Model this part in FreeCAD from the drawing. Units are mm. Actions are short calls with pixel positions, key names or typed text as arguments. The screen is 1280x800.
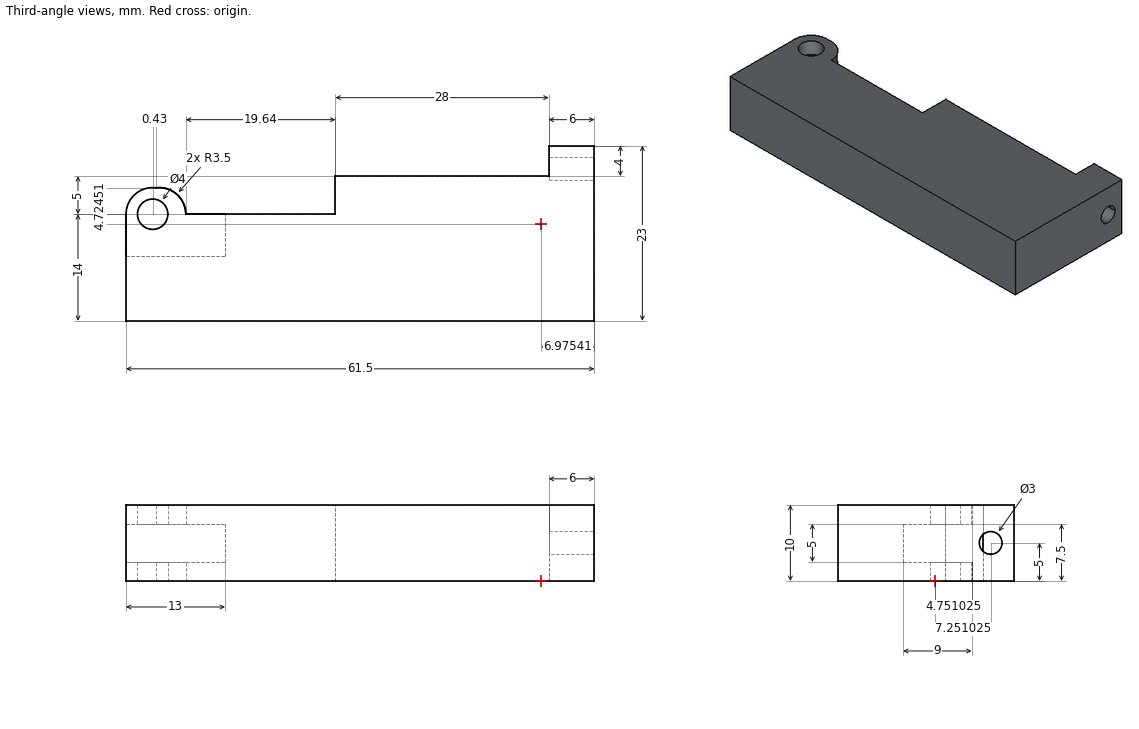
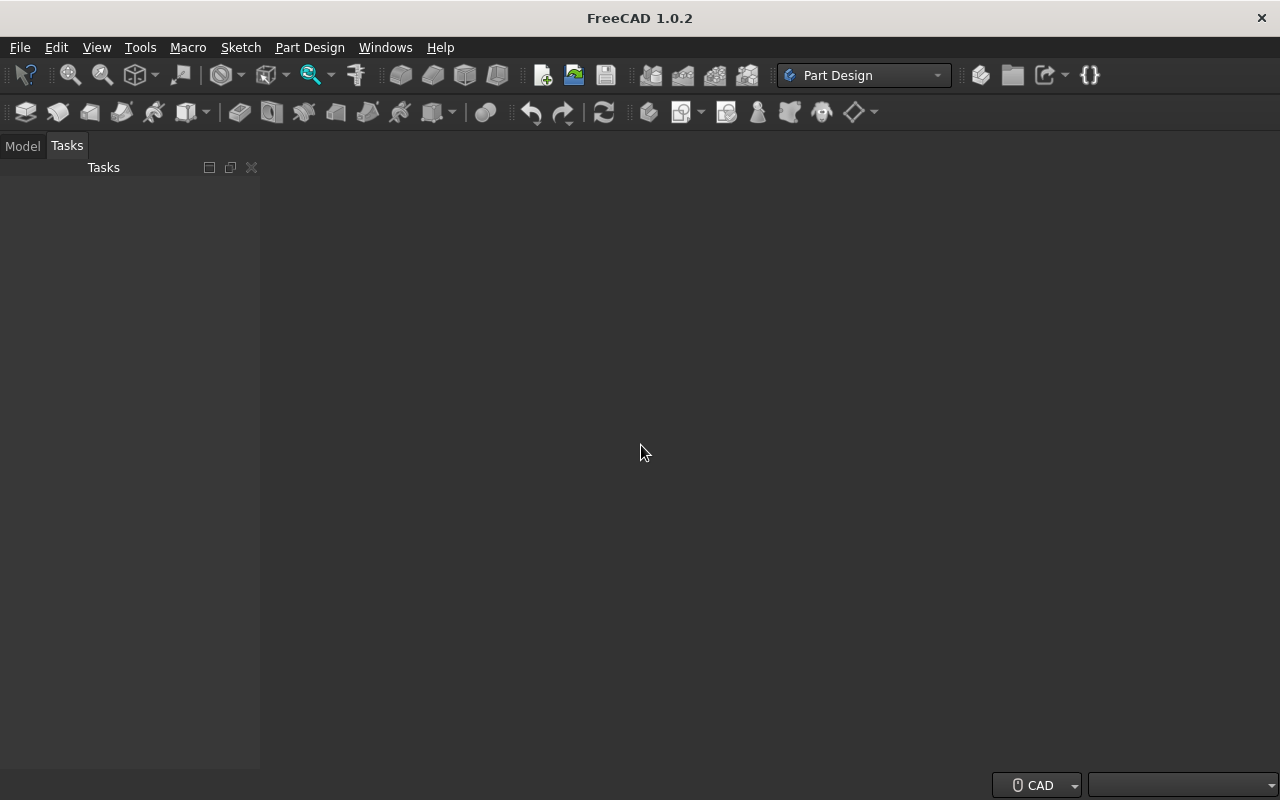
key(ctrl+n)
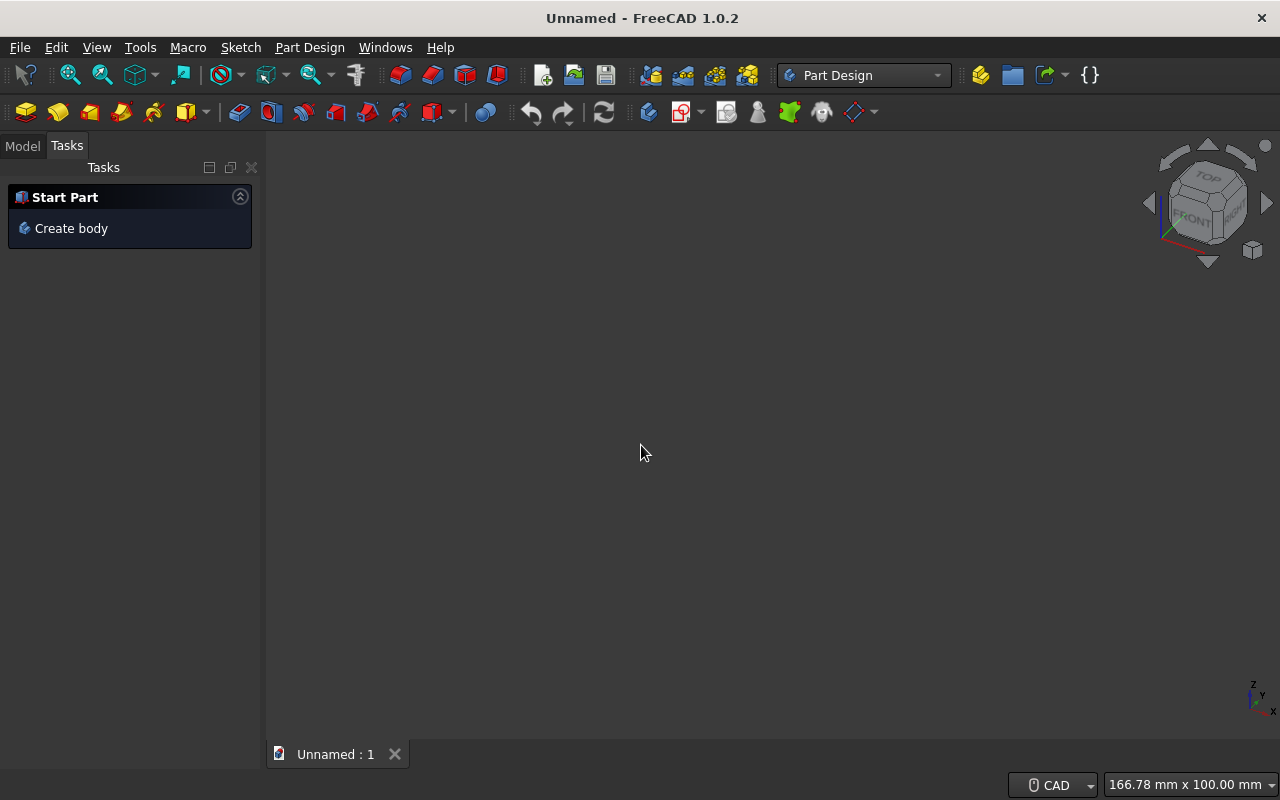
click(682, 112)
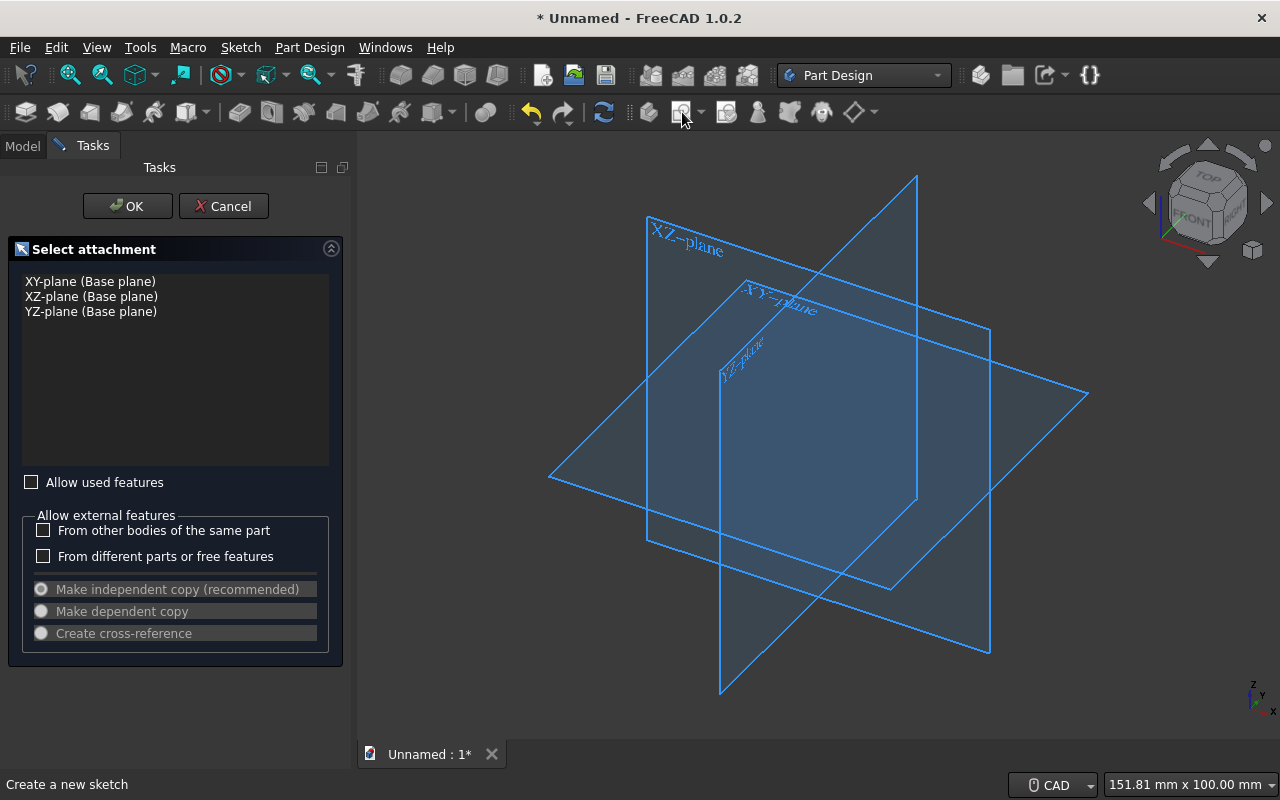
click(82, 282)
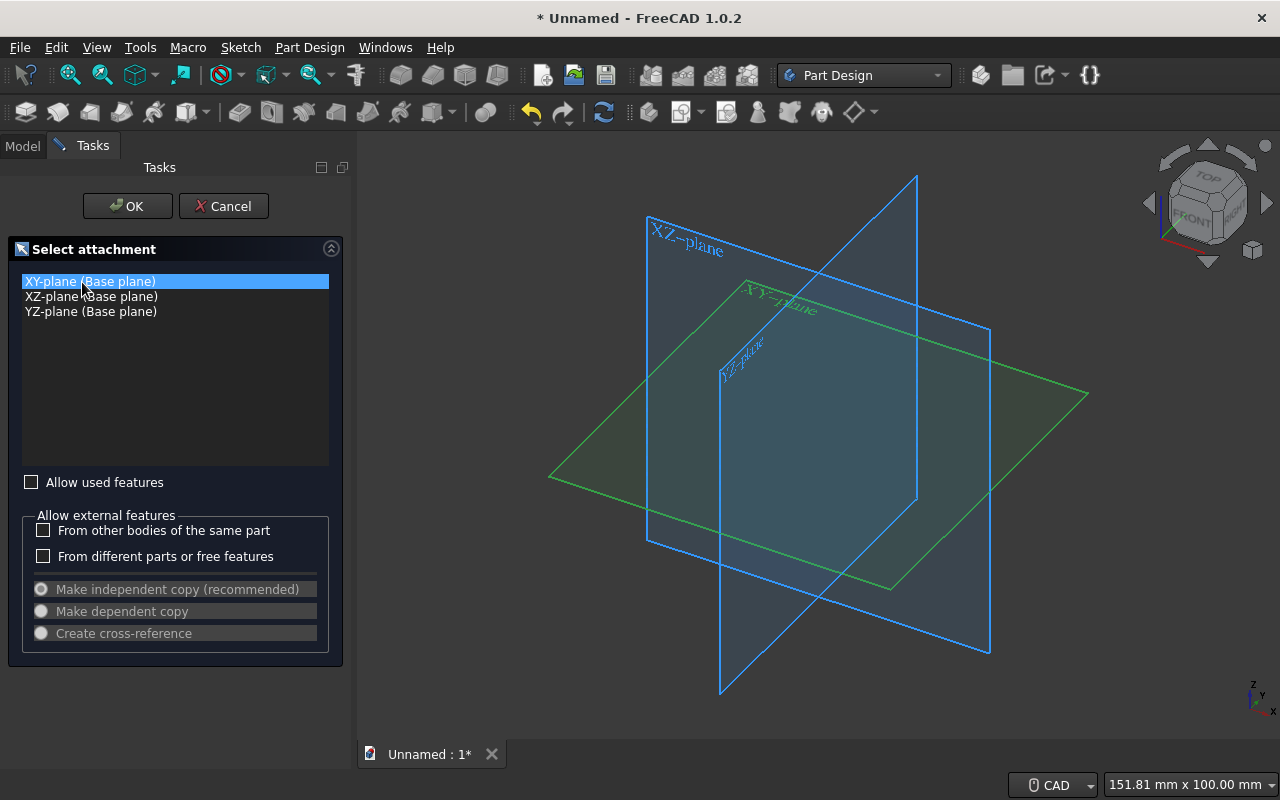
click(128, 206)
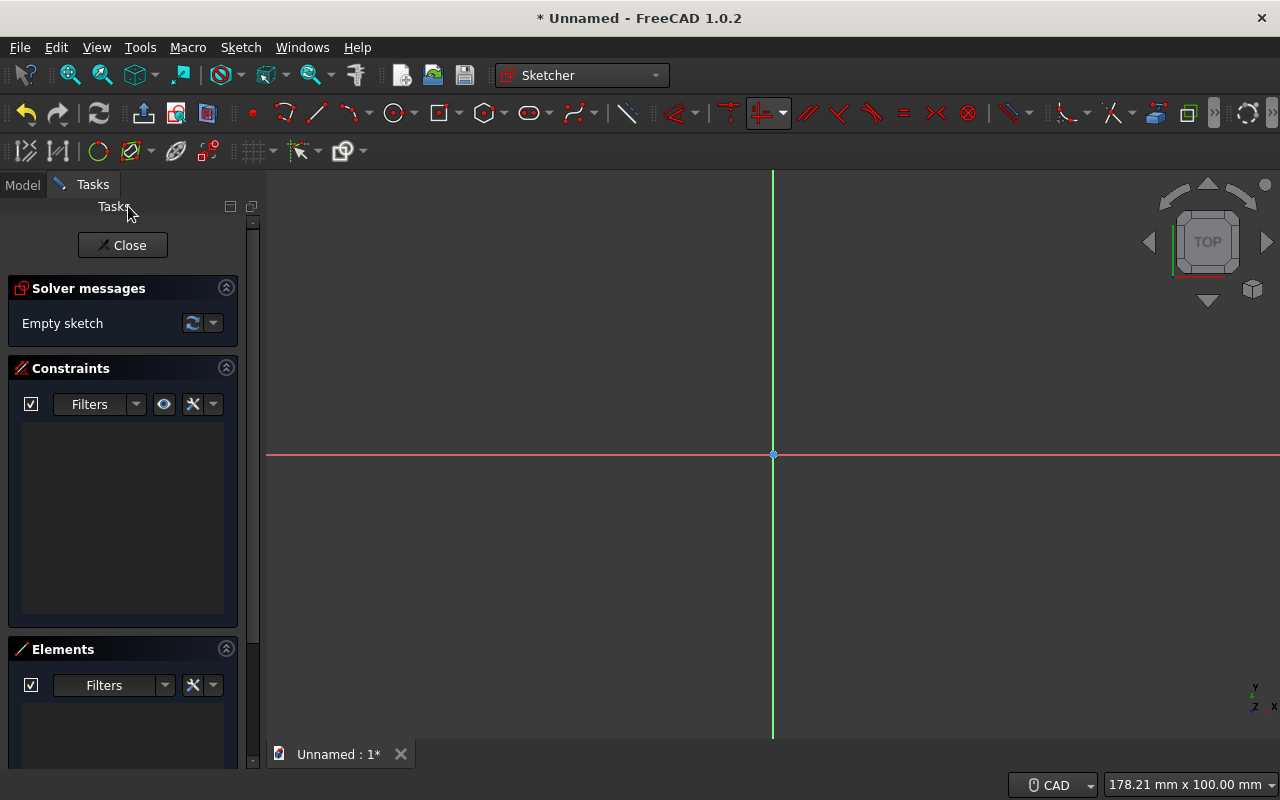
scroll(556, 470, up, 3)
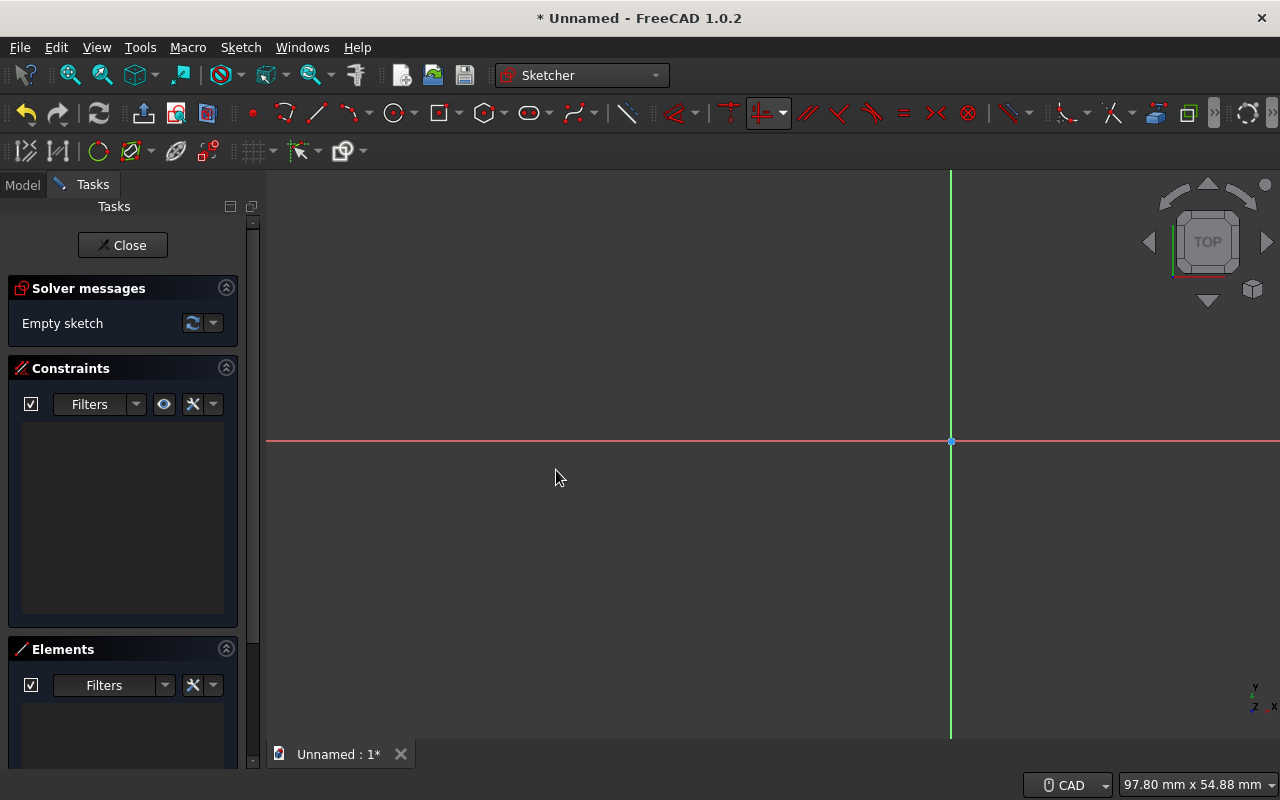
key(g)
key(m)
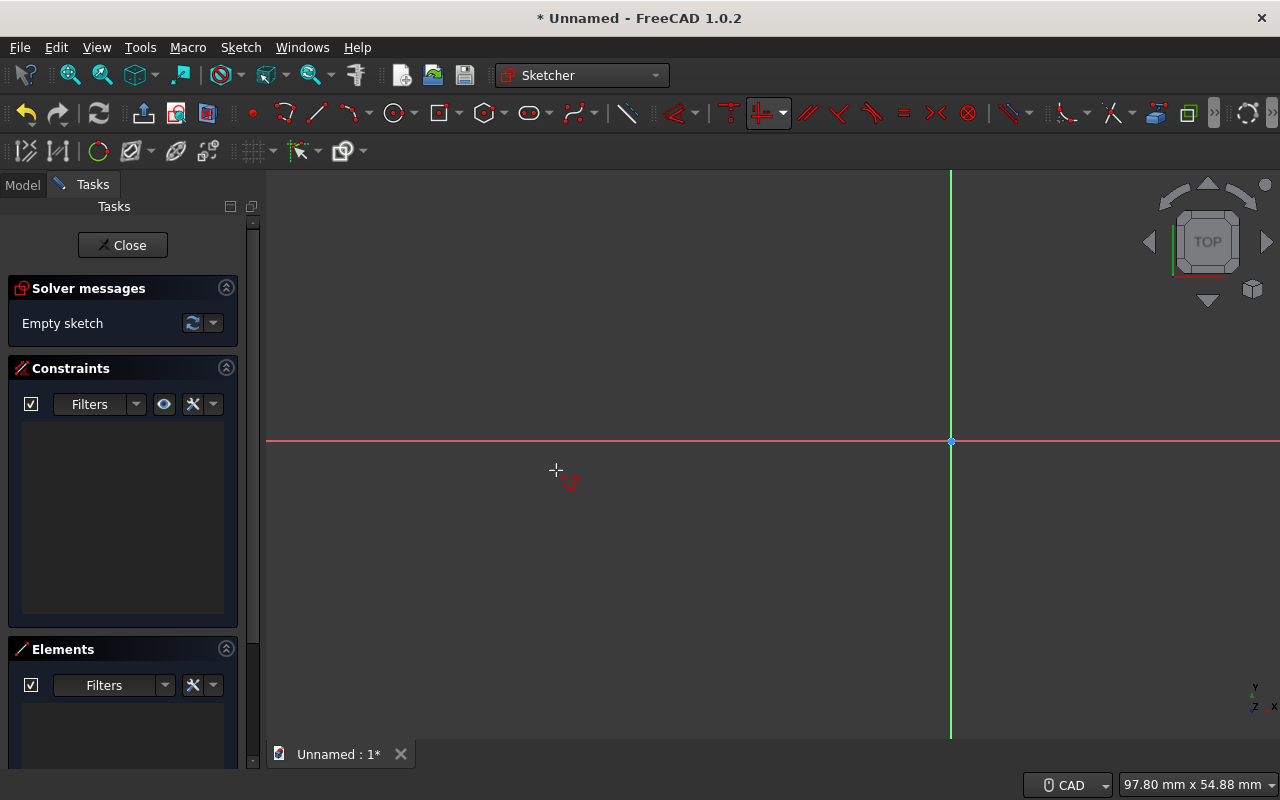
scroll(386, 428, up, 2)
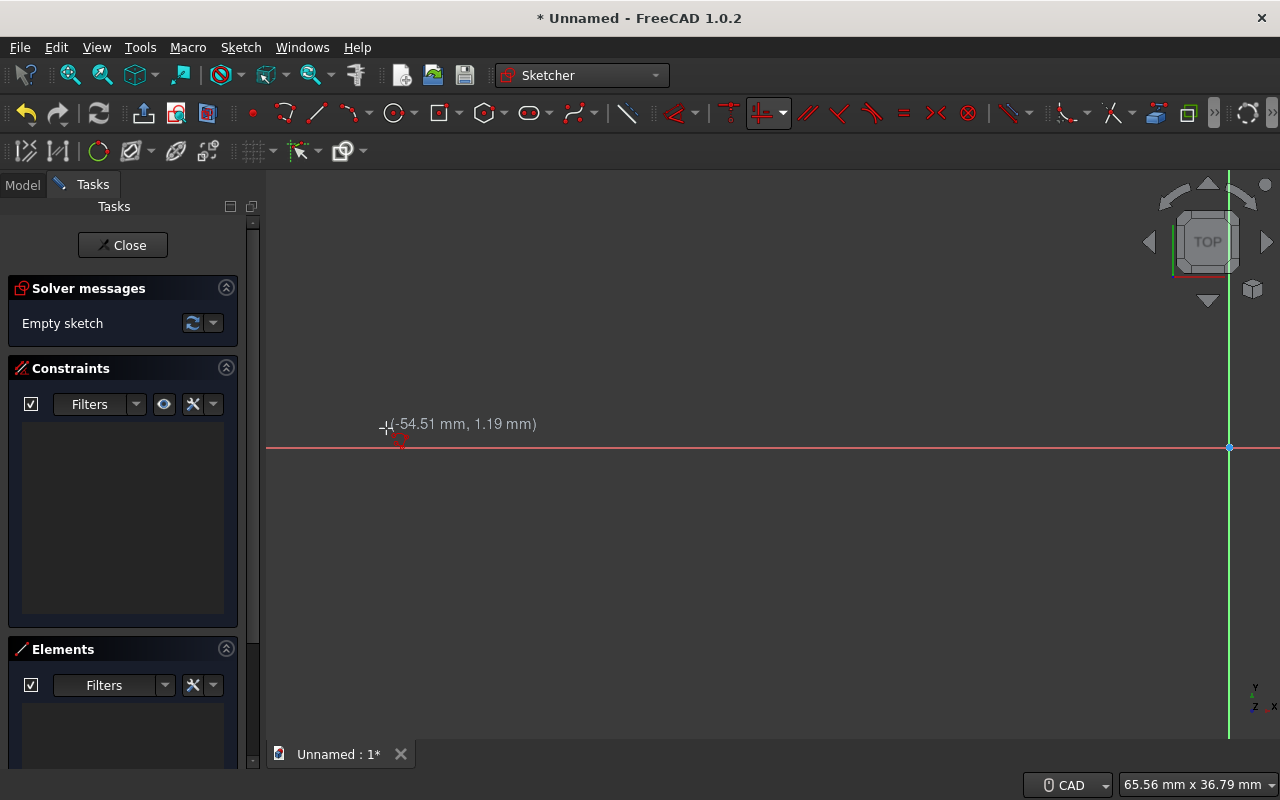
click(386, 428)
click(386, 645)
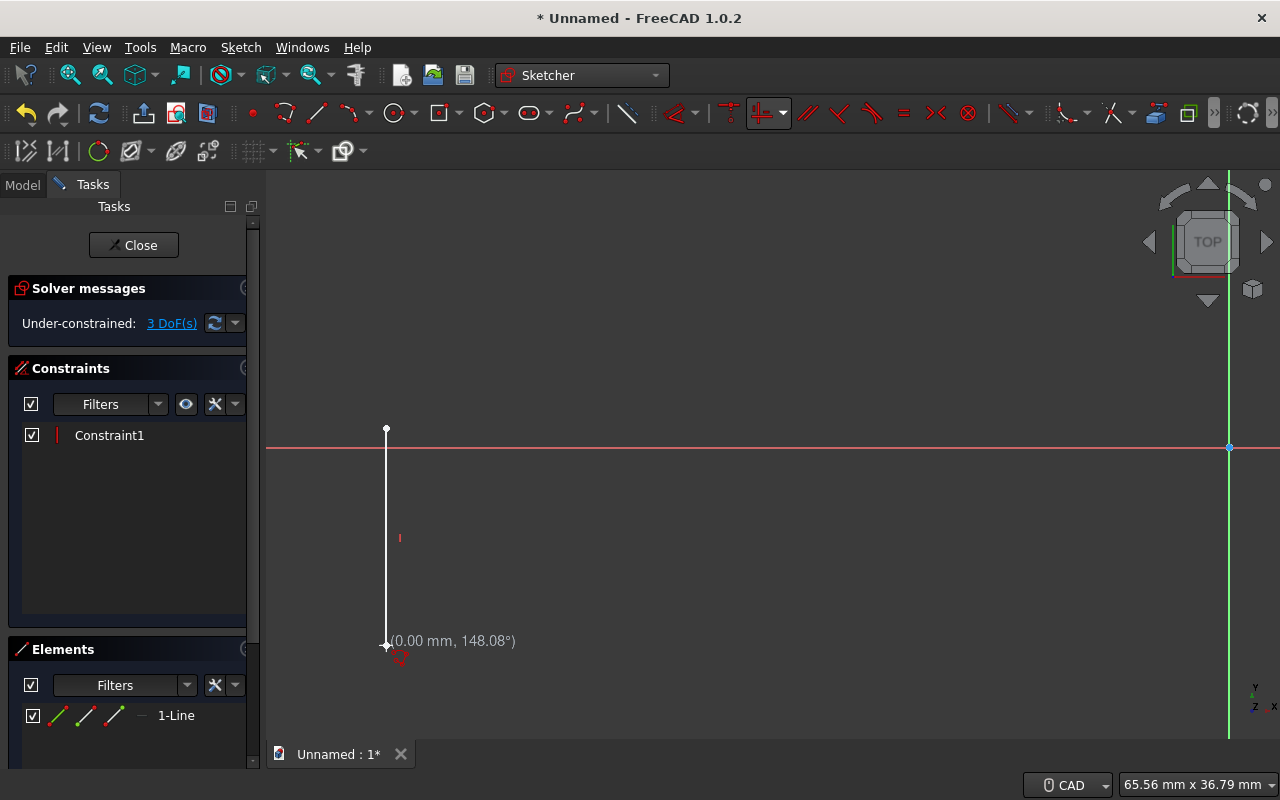
scroll(386, 429, down, 2)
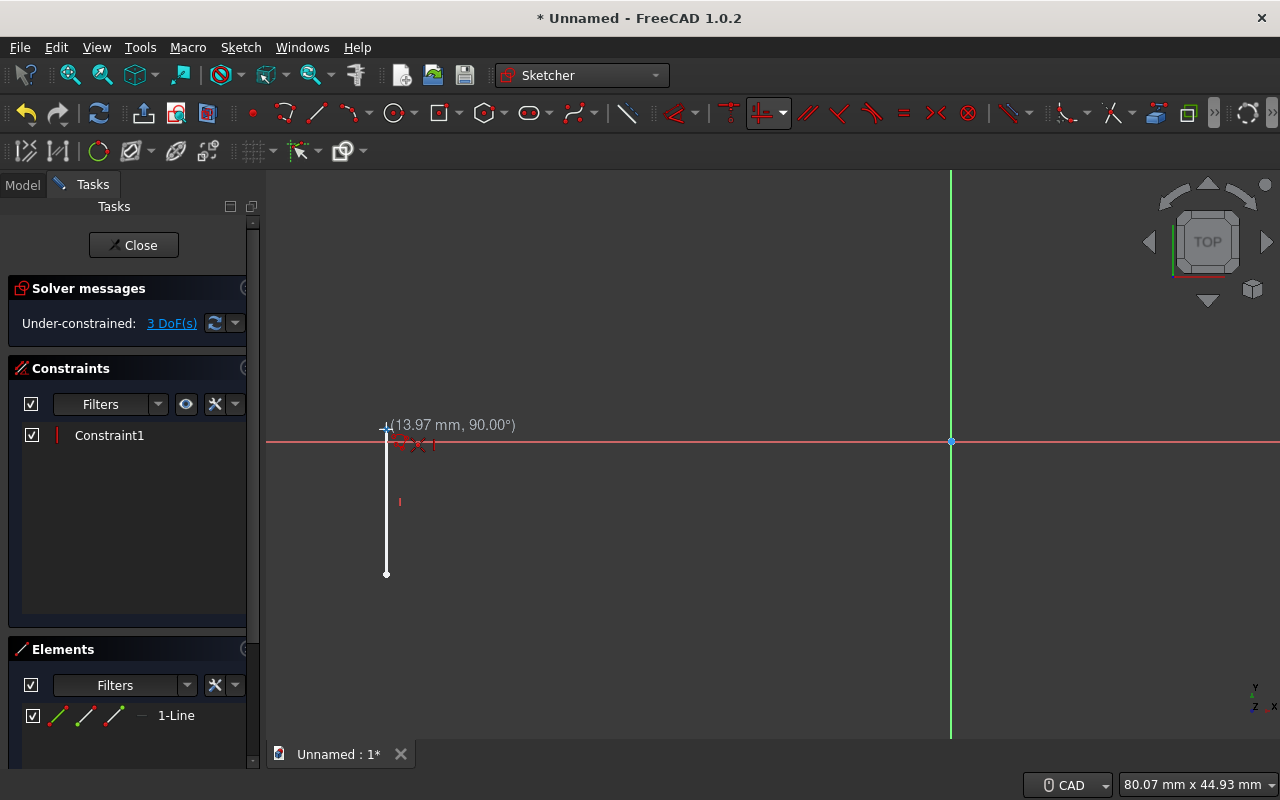
click(1023, 574)
click(1023, 335)